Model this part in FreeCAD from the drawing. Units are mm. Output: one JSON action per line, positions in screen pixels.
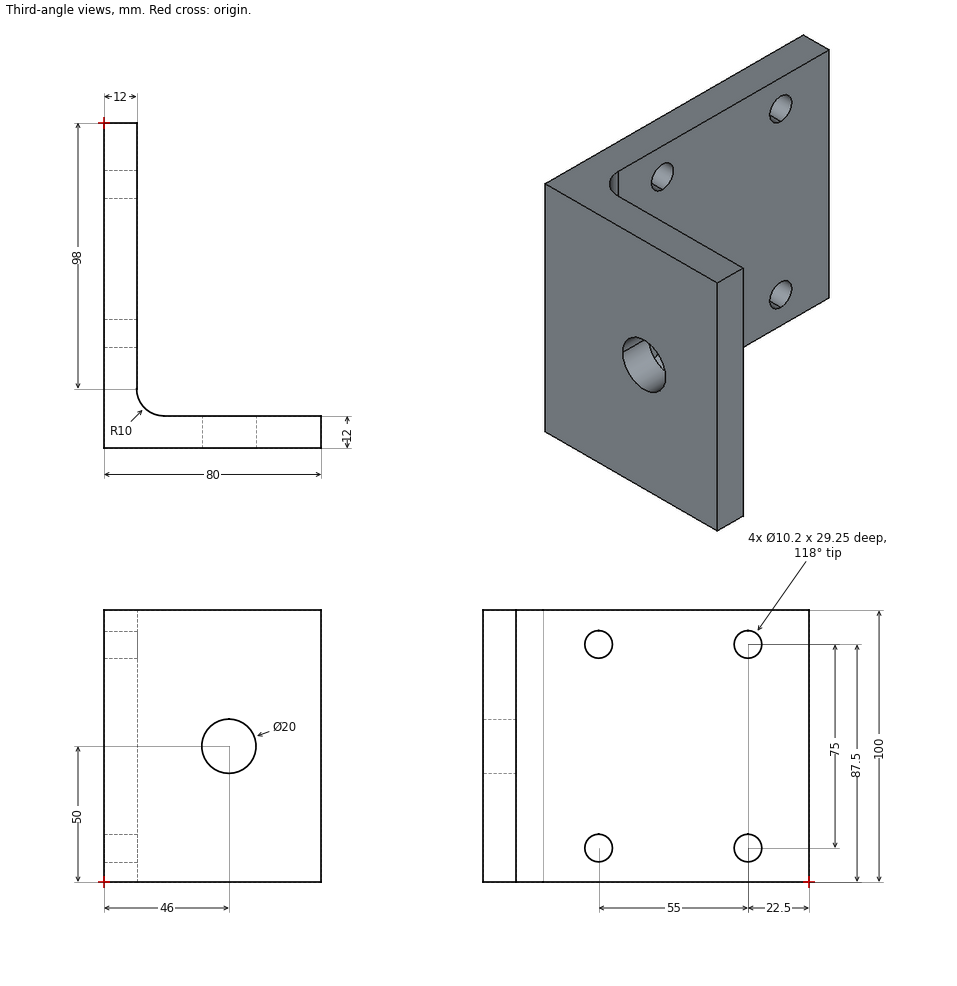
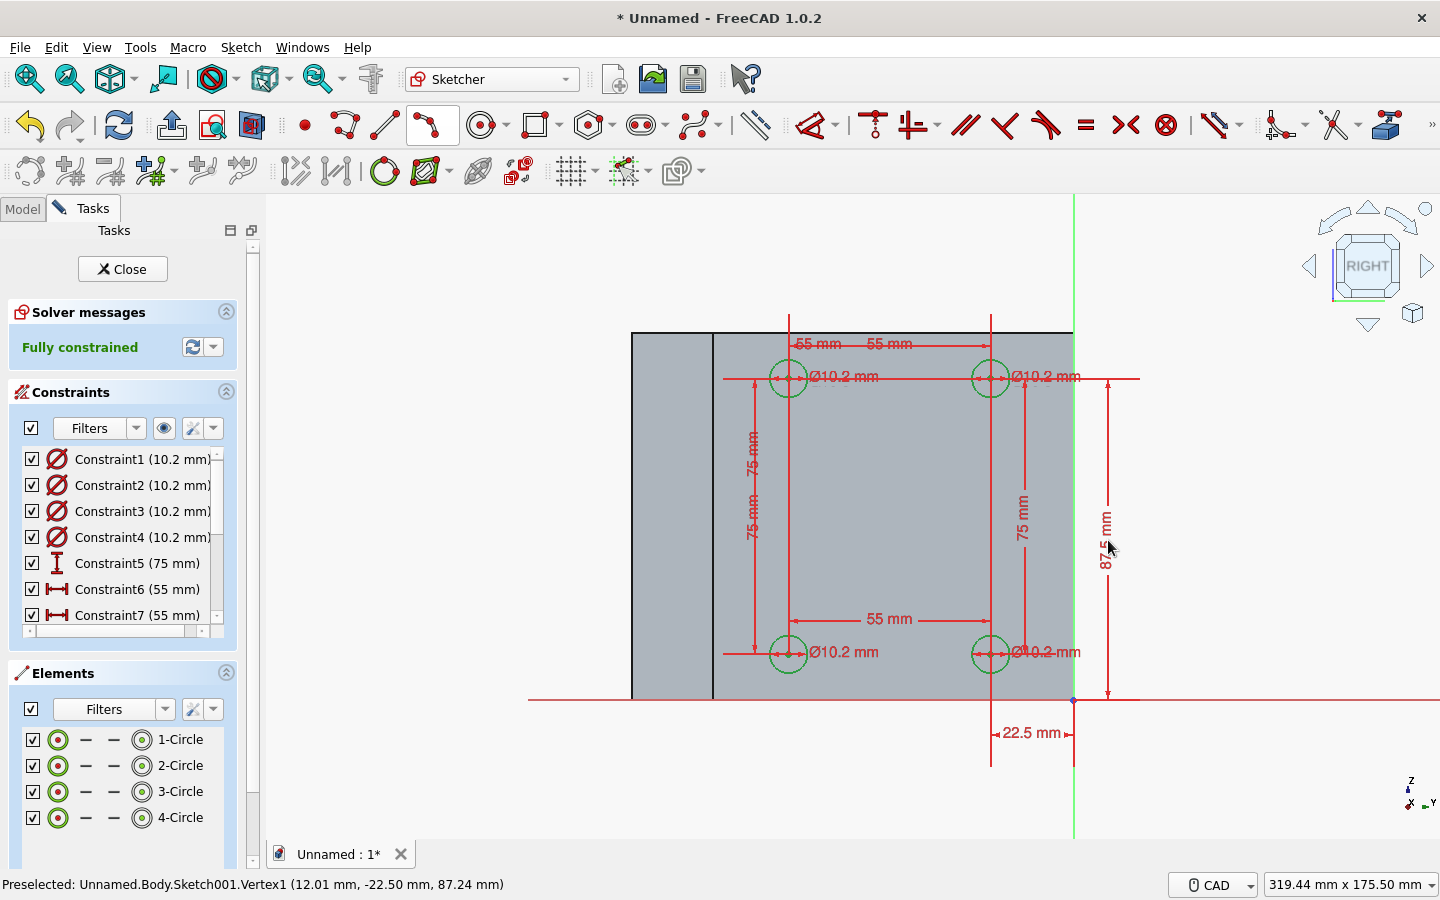
{"action": "left_click", "coordinate": [123, 269]}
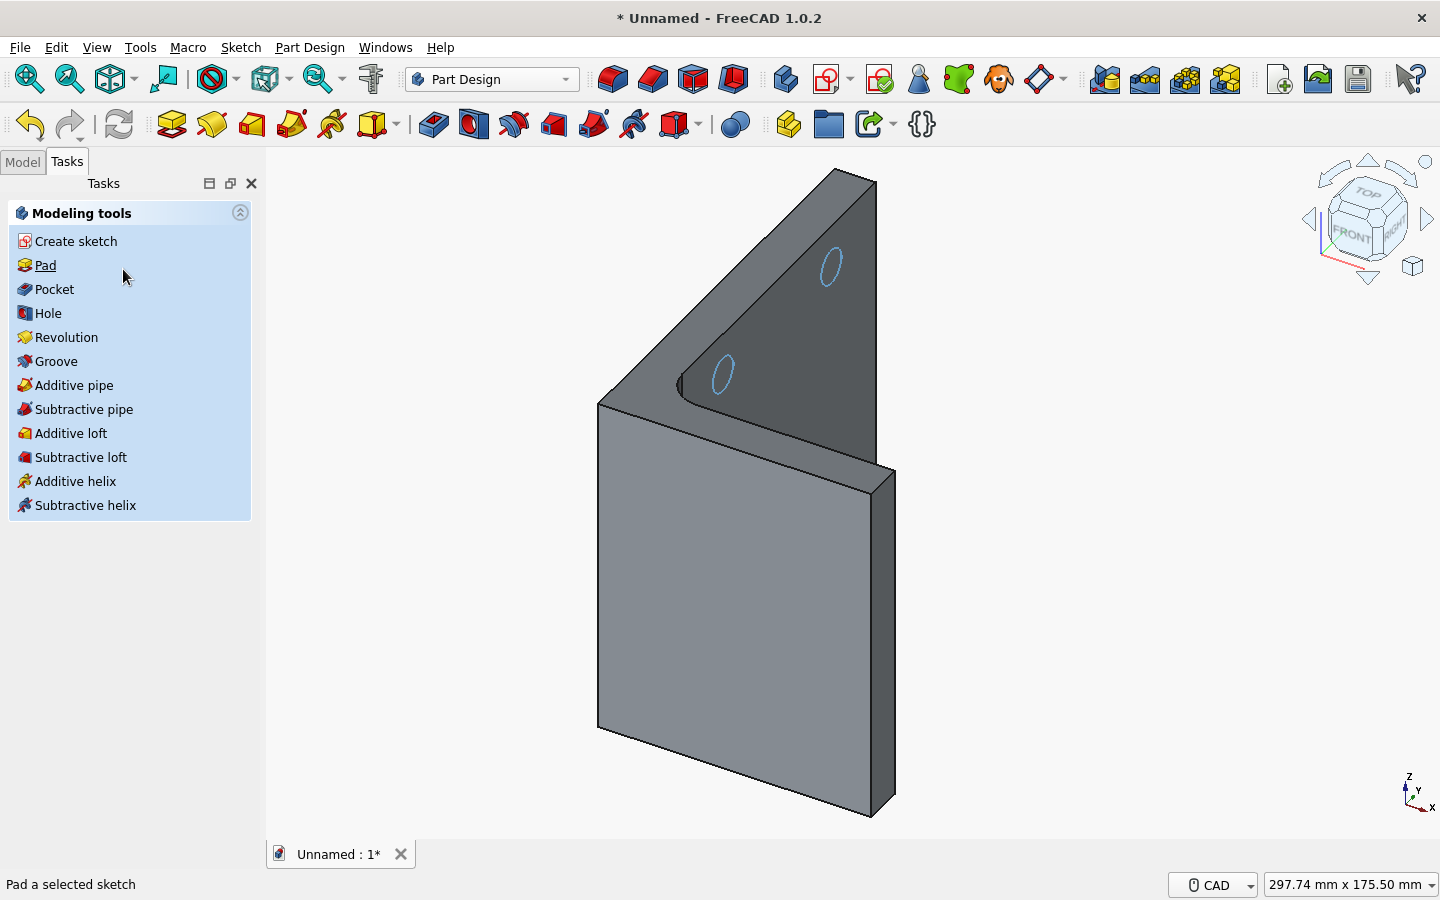
{"action": "left_click", "coordinate": [474, 124]}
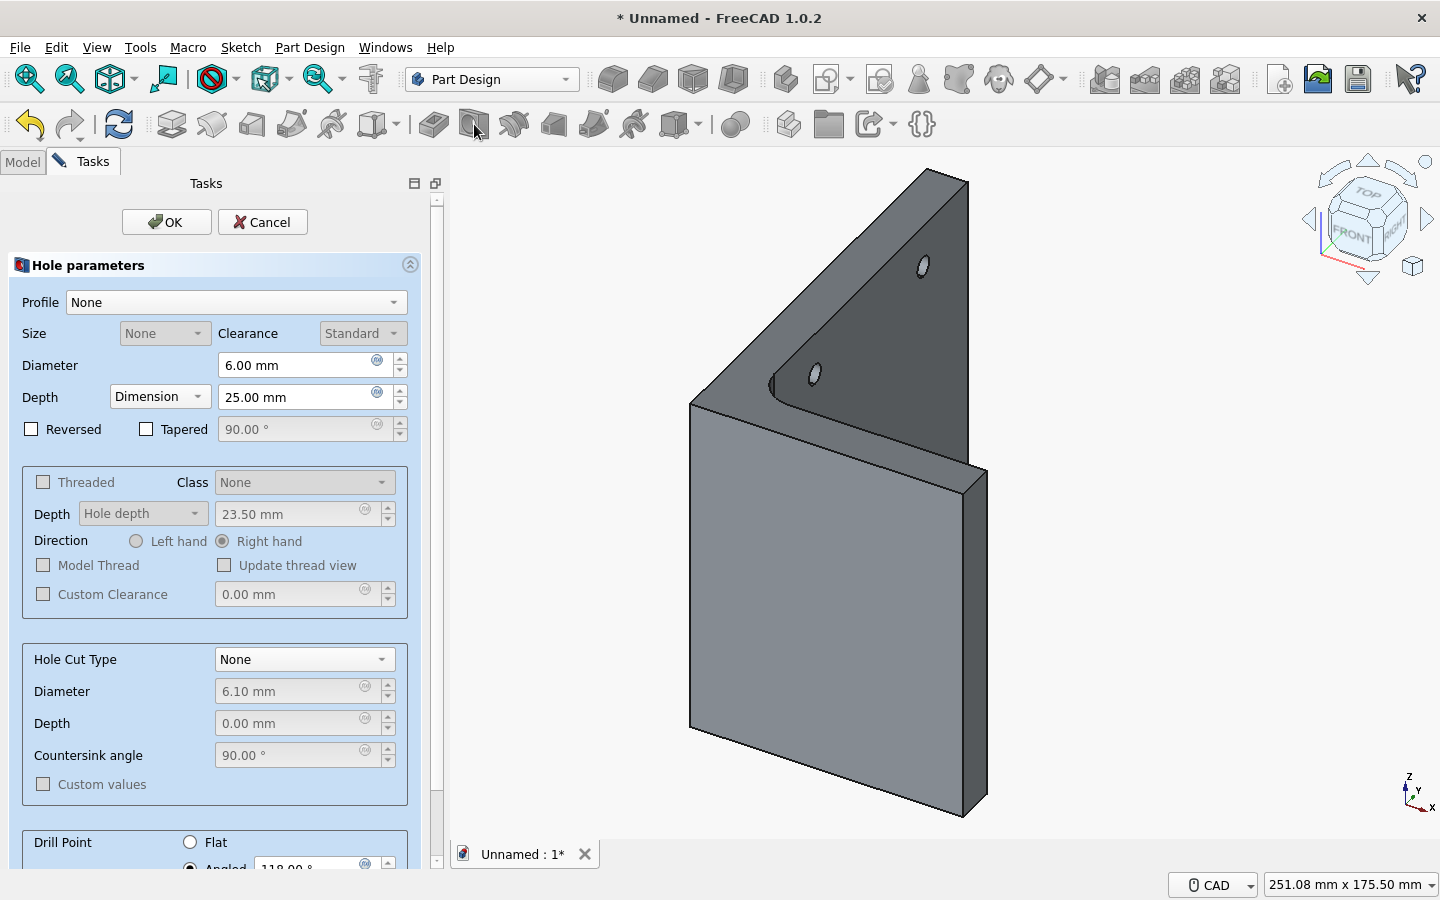
{"action": "triple_click", "coordinate": [305, 365]}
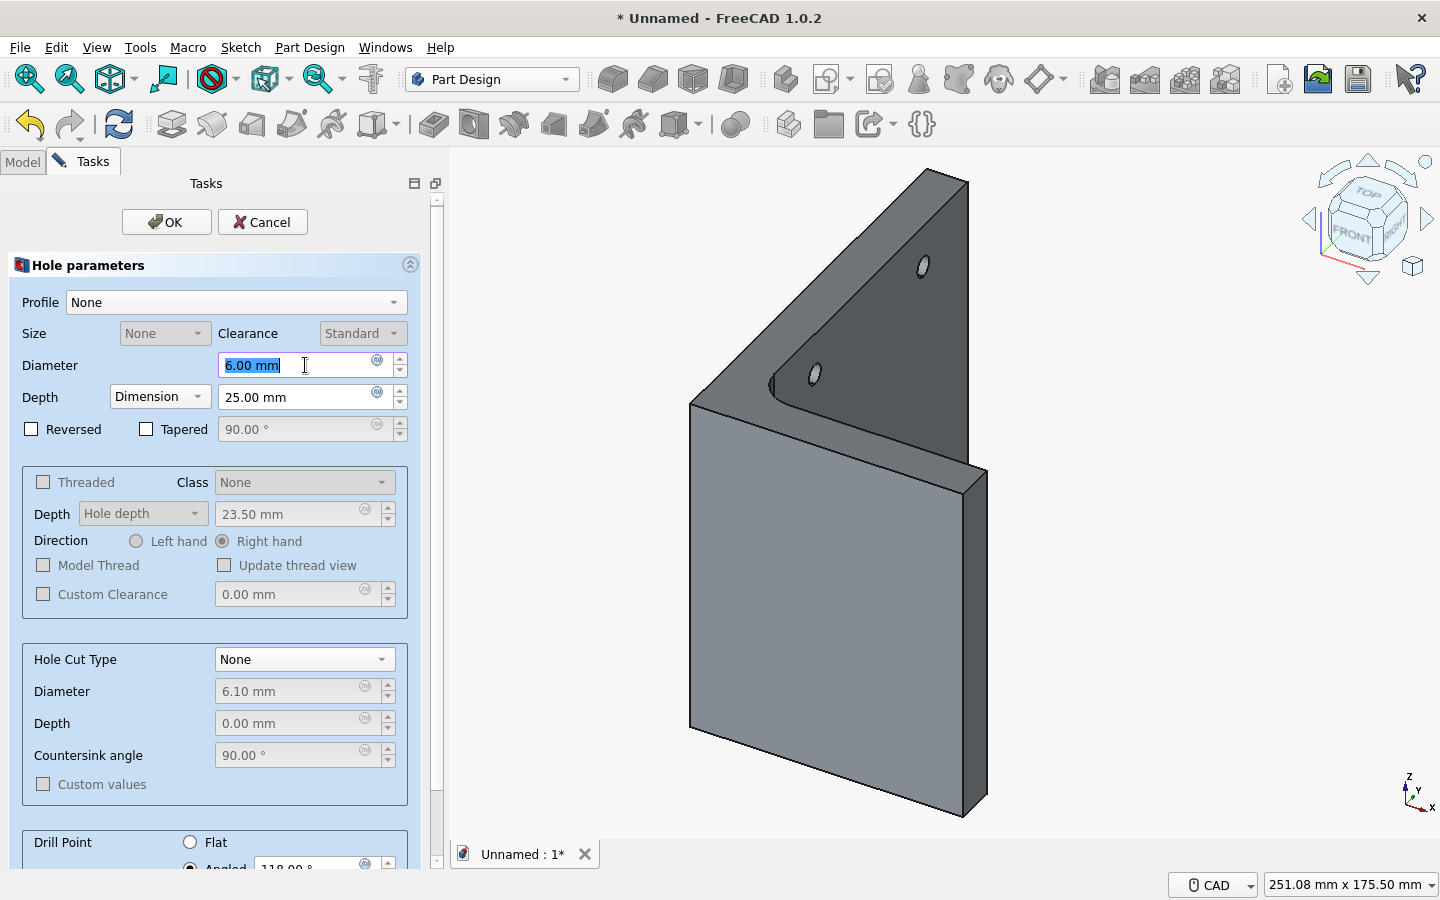
{"action": "type", "text": "10.2"}
{"action": "key", "text": "Tab"}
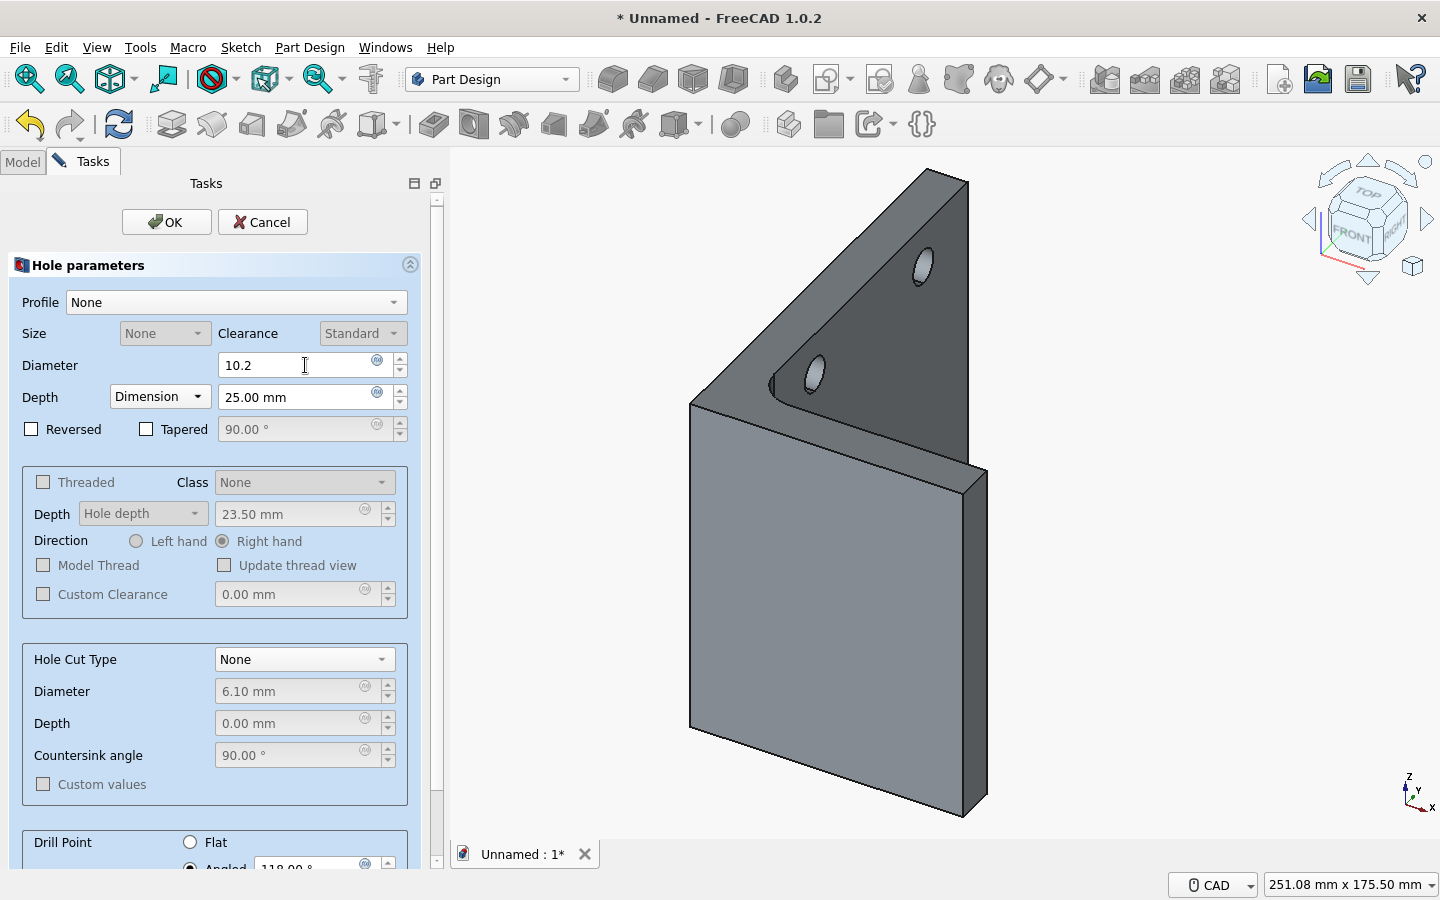
{"action": "triple_click", "coordinate": [305, 397]}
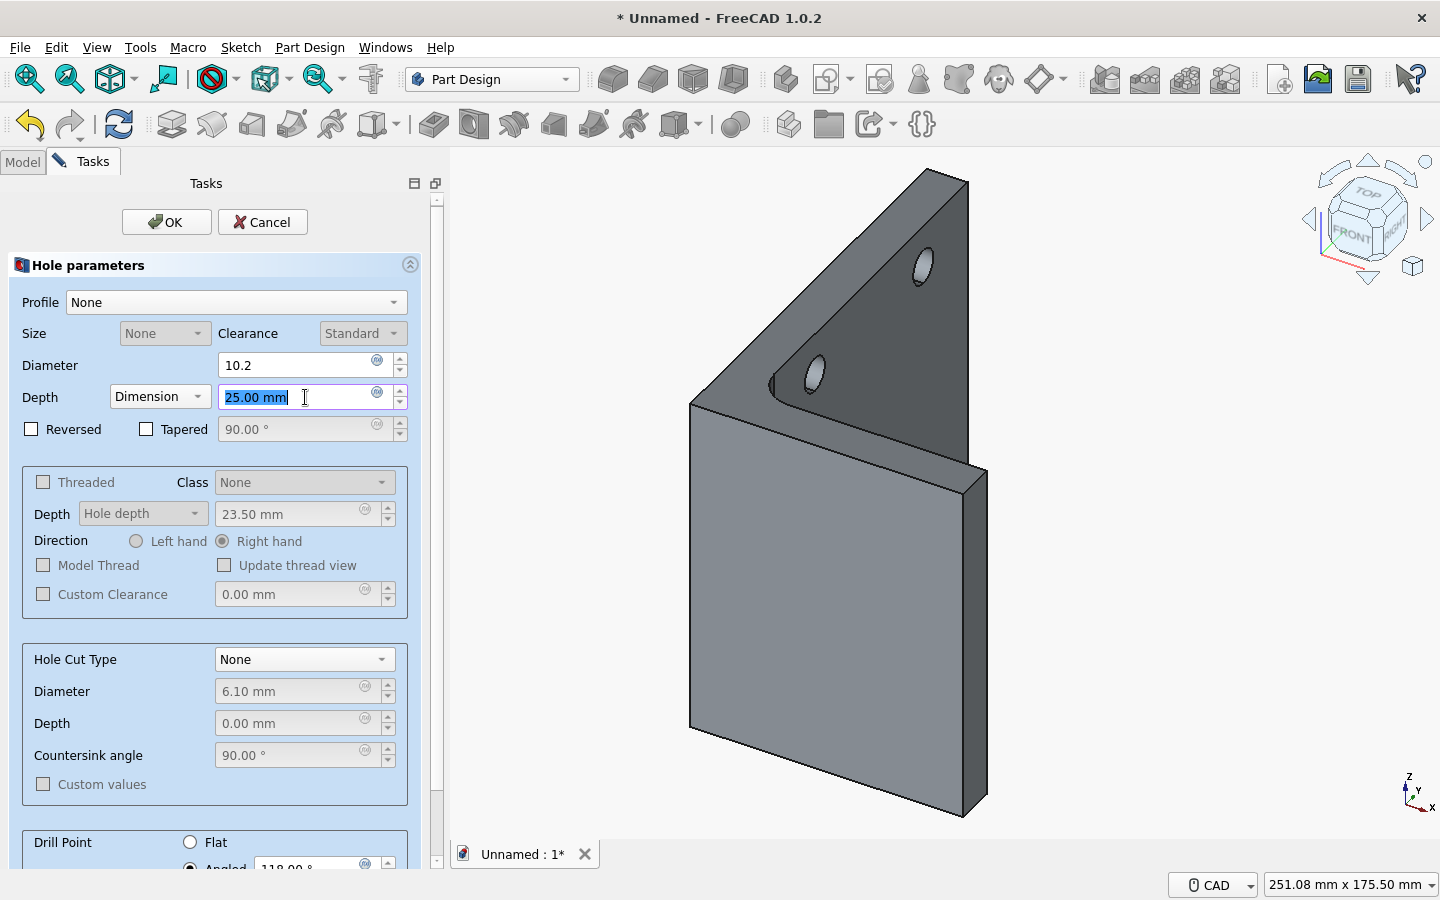
{"action": "type", "text": "29.25"}
{"action": "key", "text": "Tab"}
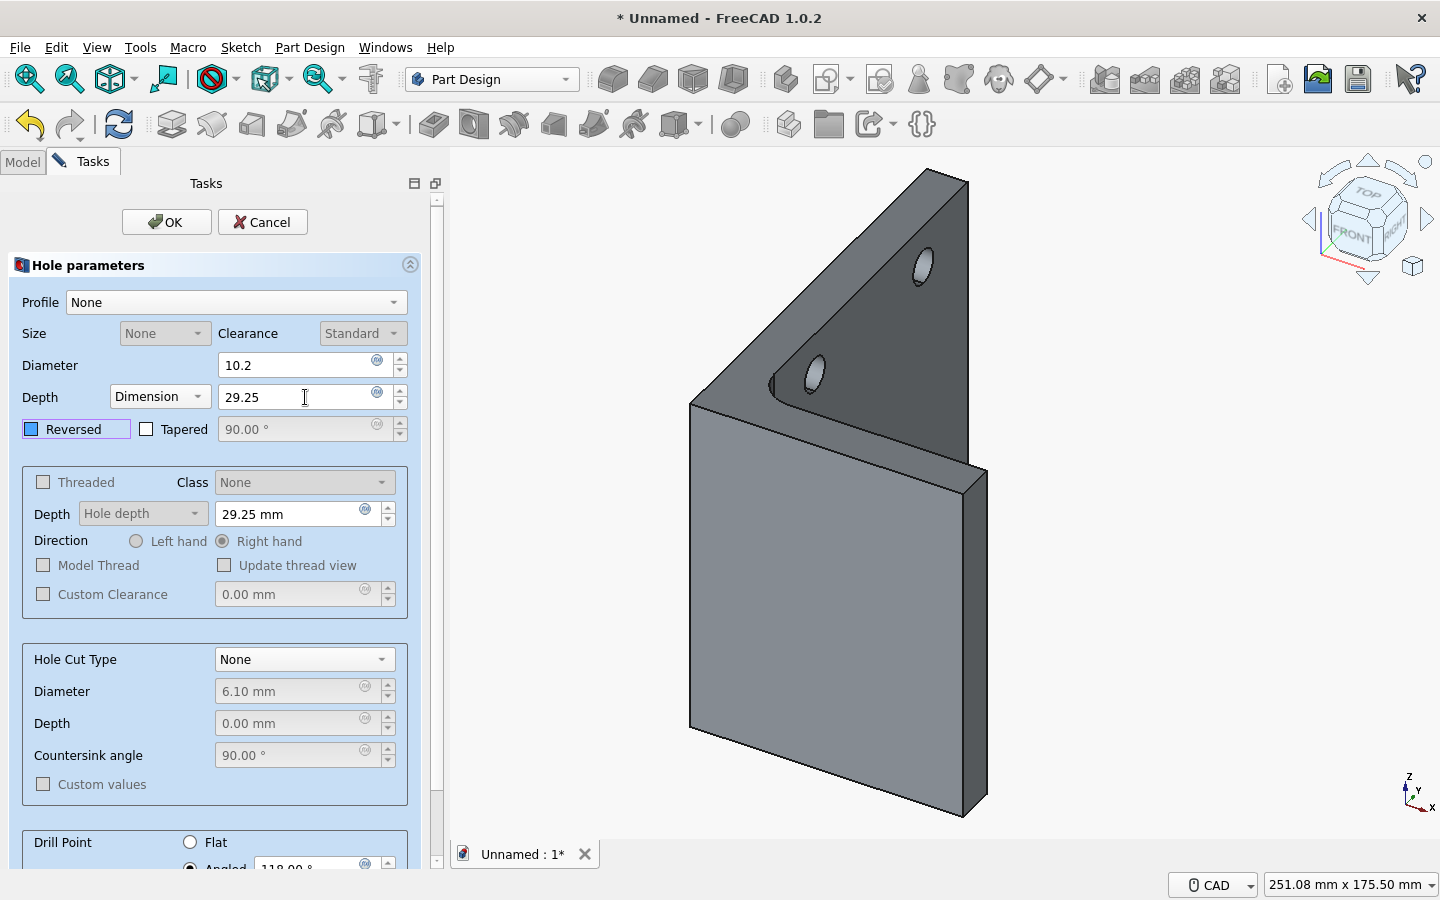
{"action": "left_click", "coordinate": [167, 222]}